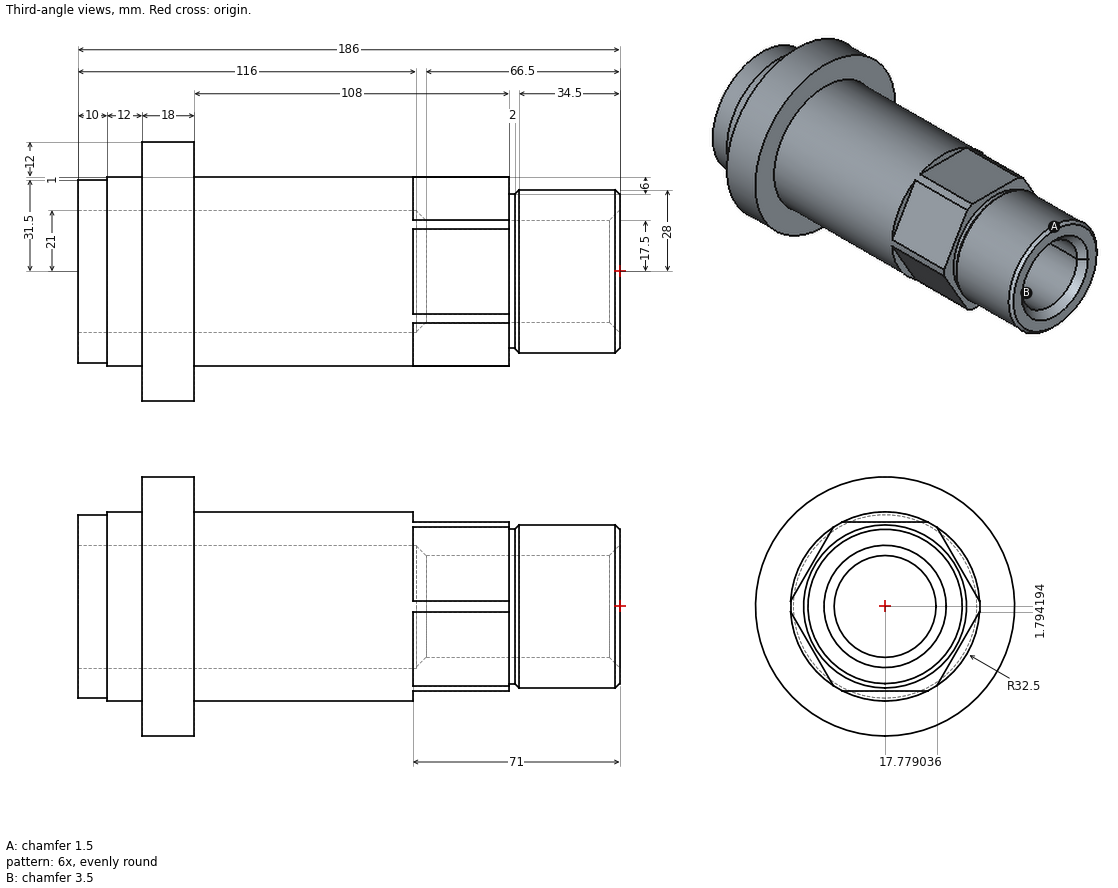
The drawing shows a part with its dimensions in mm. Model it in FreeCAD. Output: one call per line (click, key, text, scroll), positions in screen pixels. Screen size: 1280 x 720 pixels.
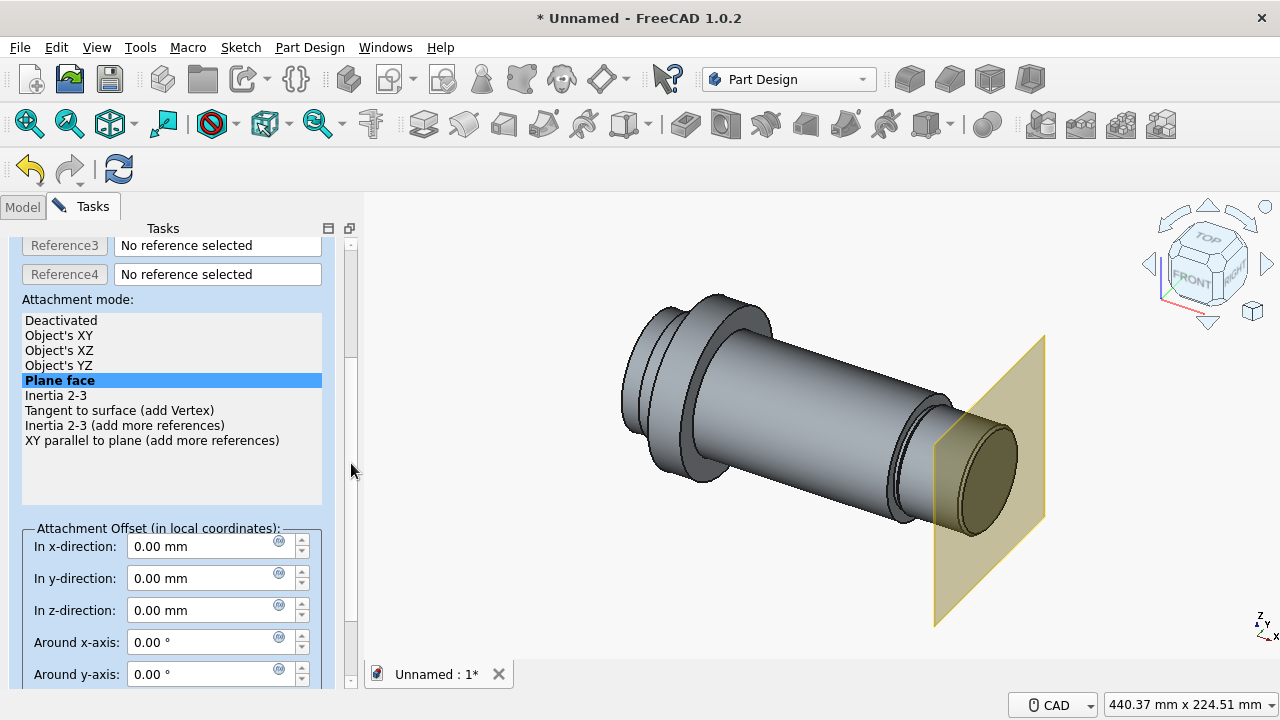
triple_click(210, 610)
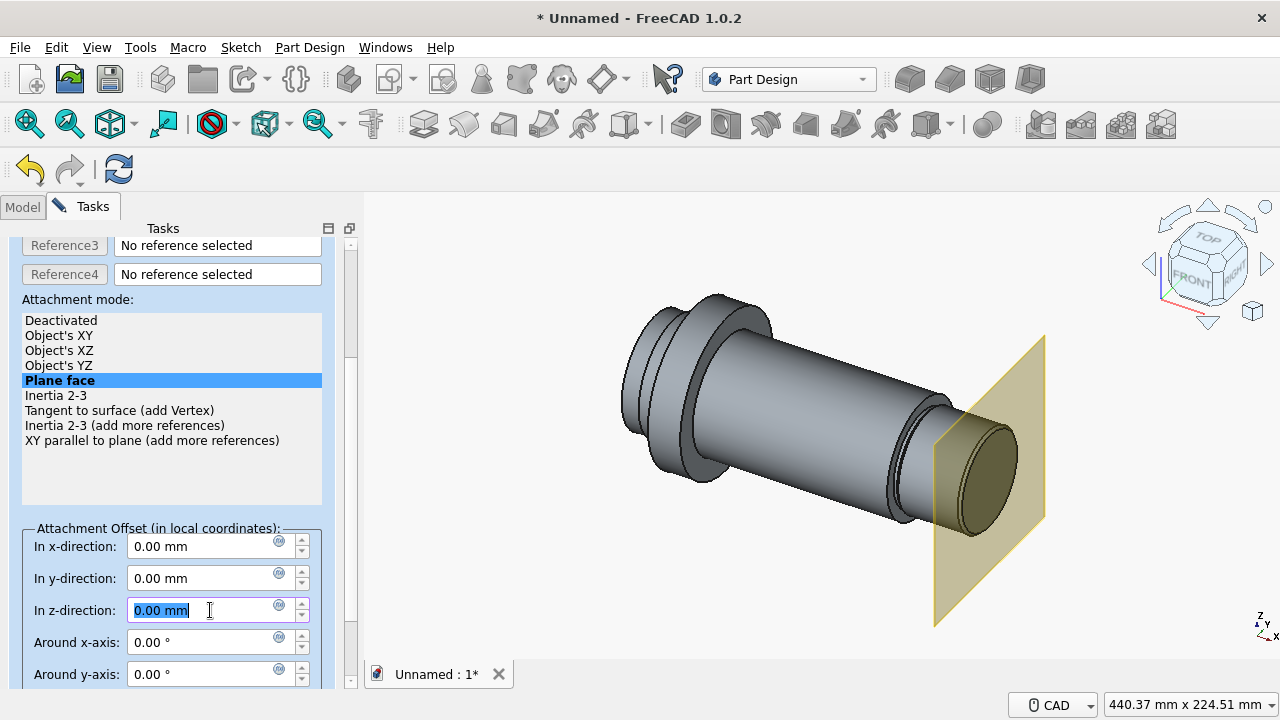
text(-71)
key(Tab)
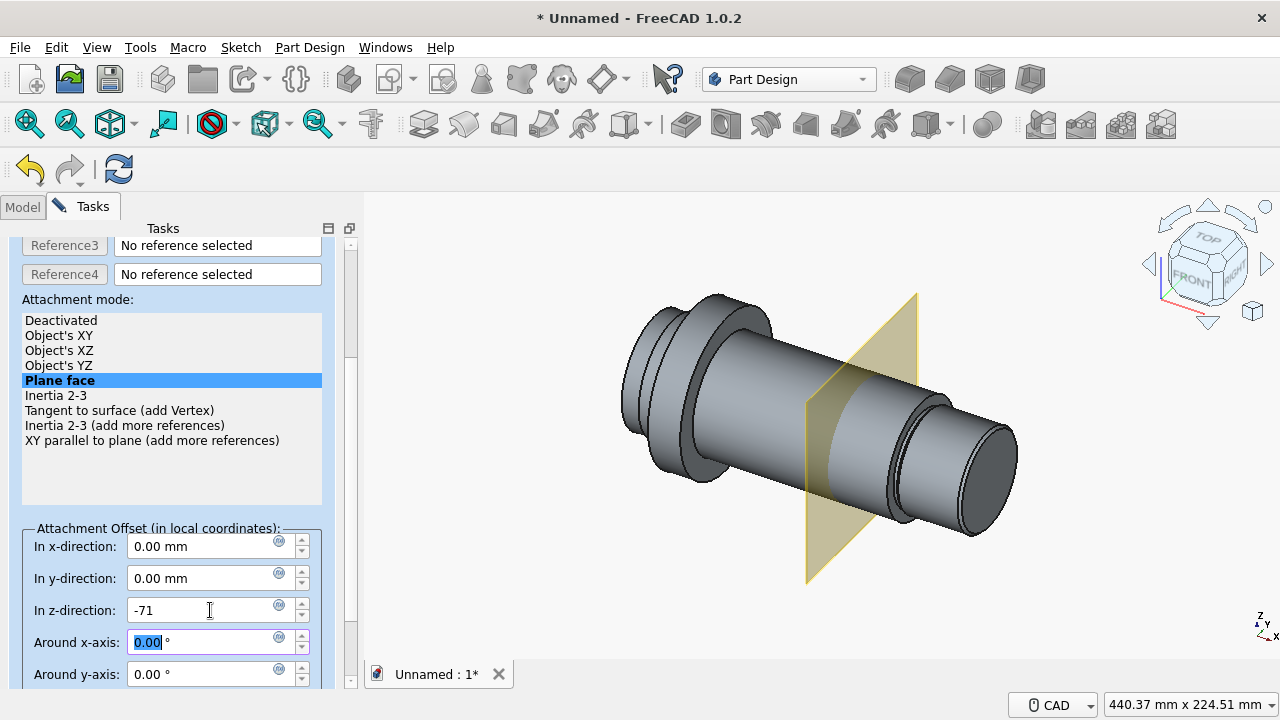
scroll(351, 463, up, 4)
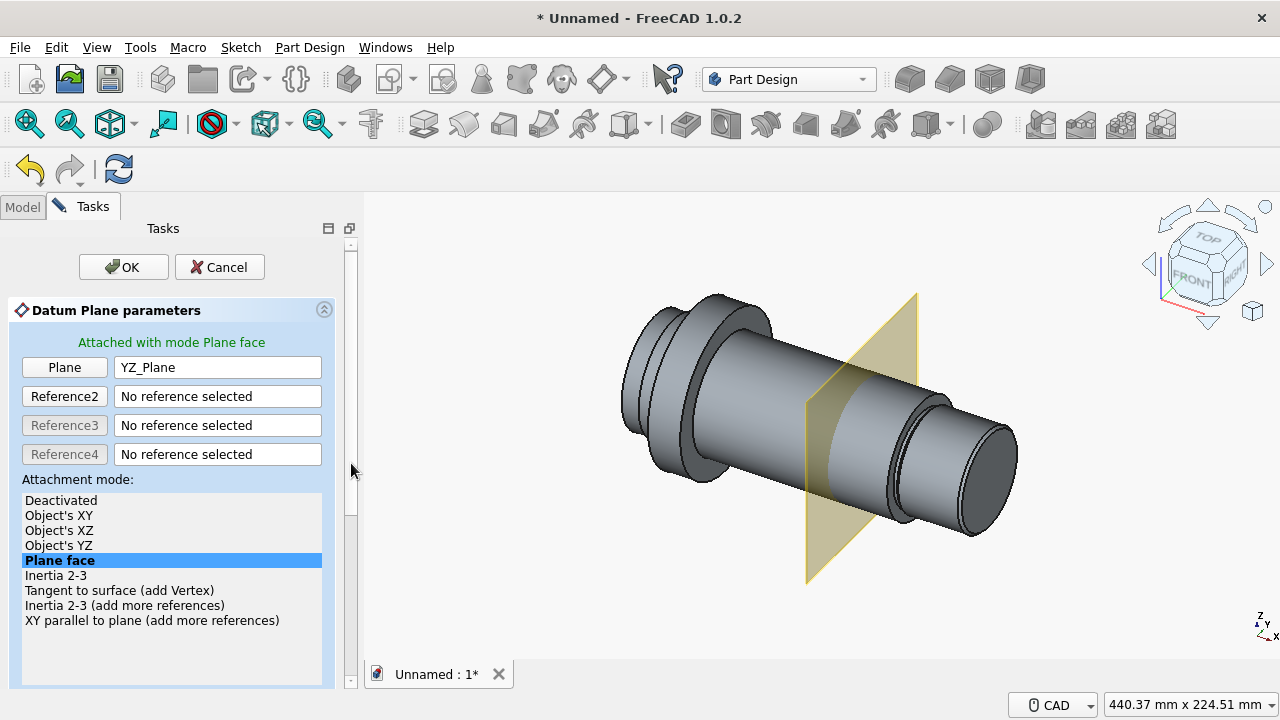
click(124, 267)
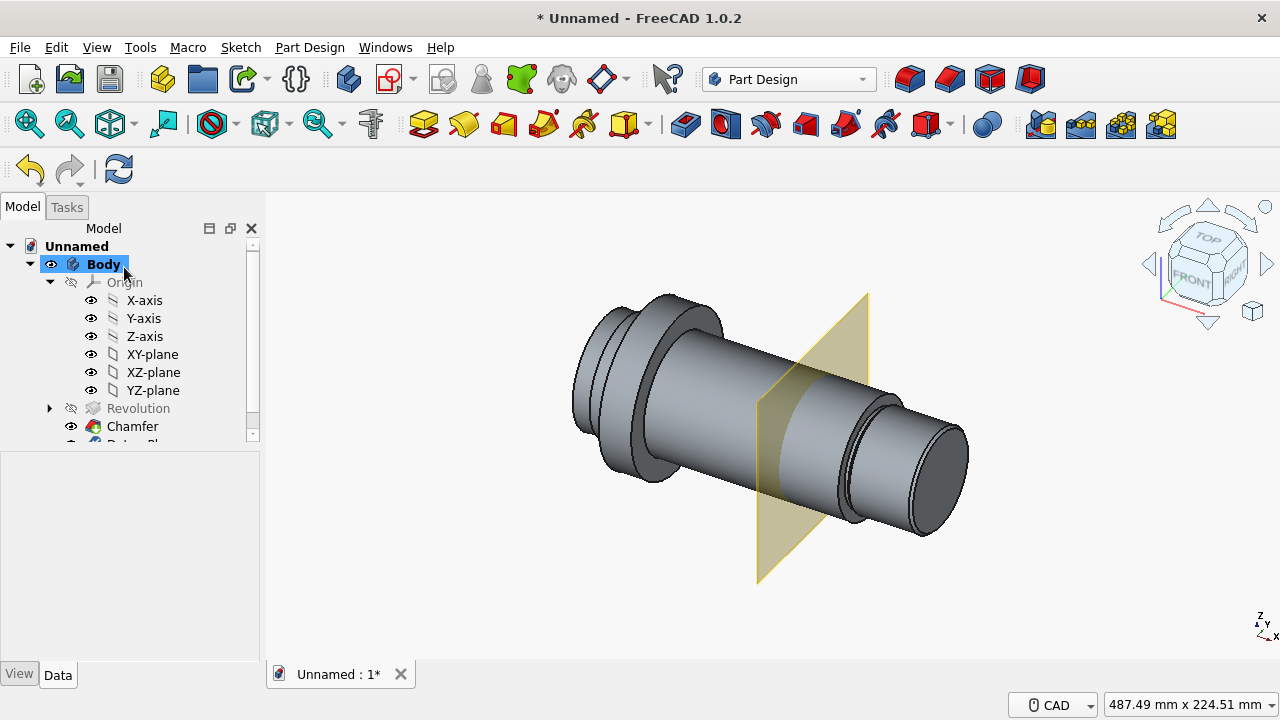
scroll(100, 332, down, 3)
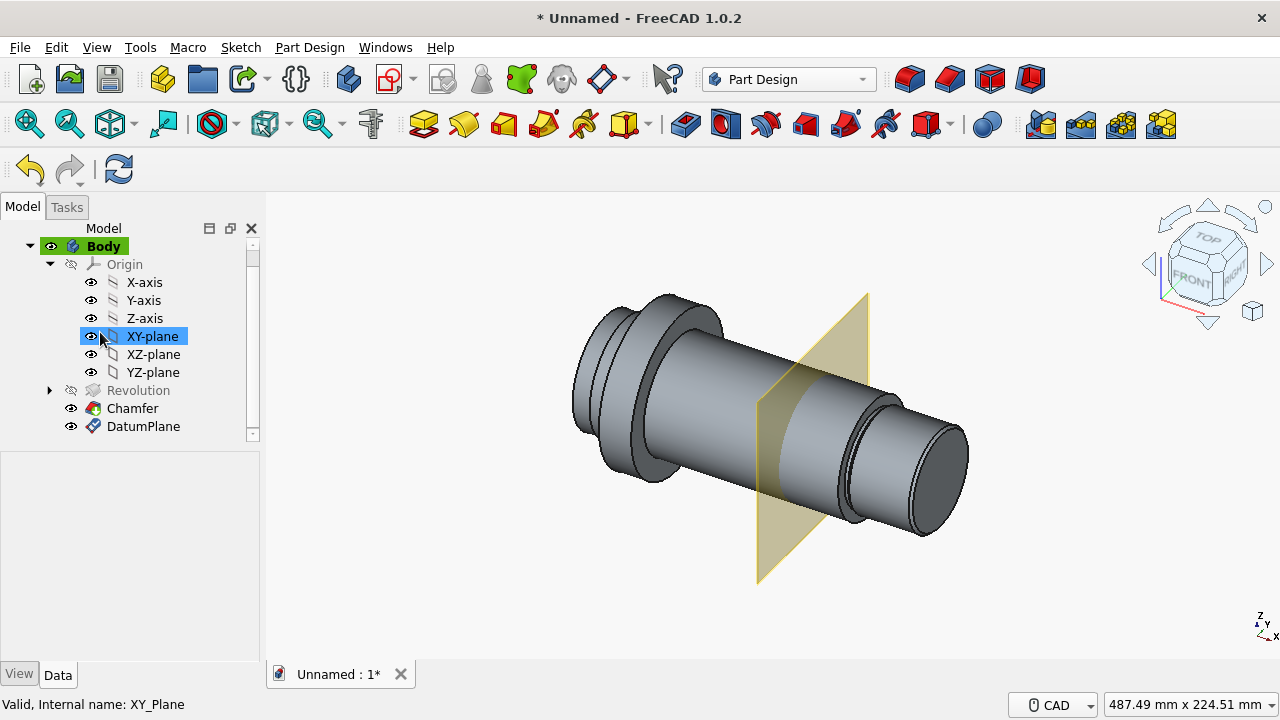
click(116, 426)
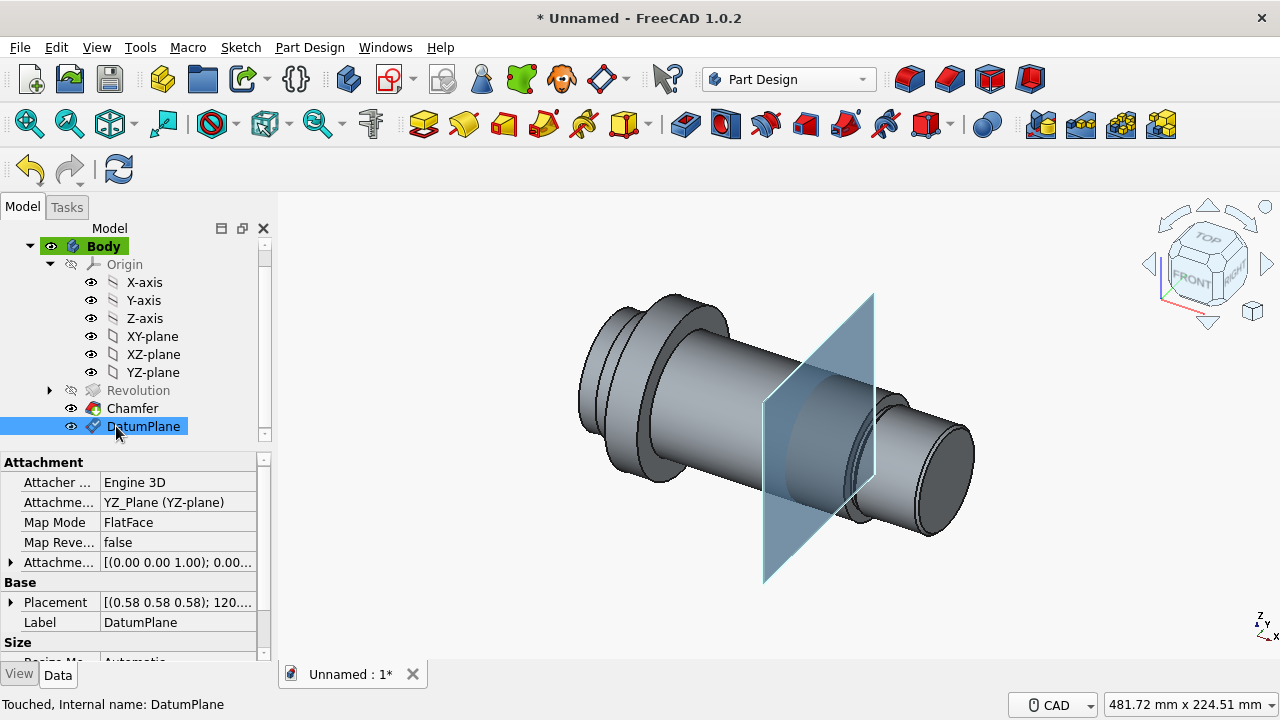
click(390, 80)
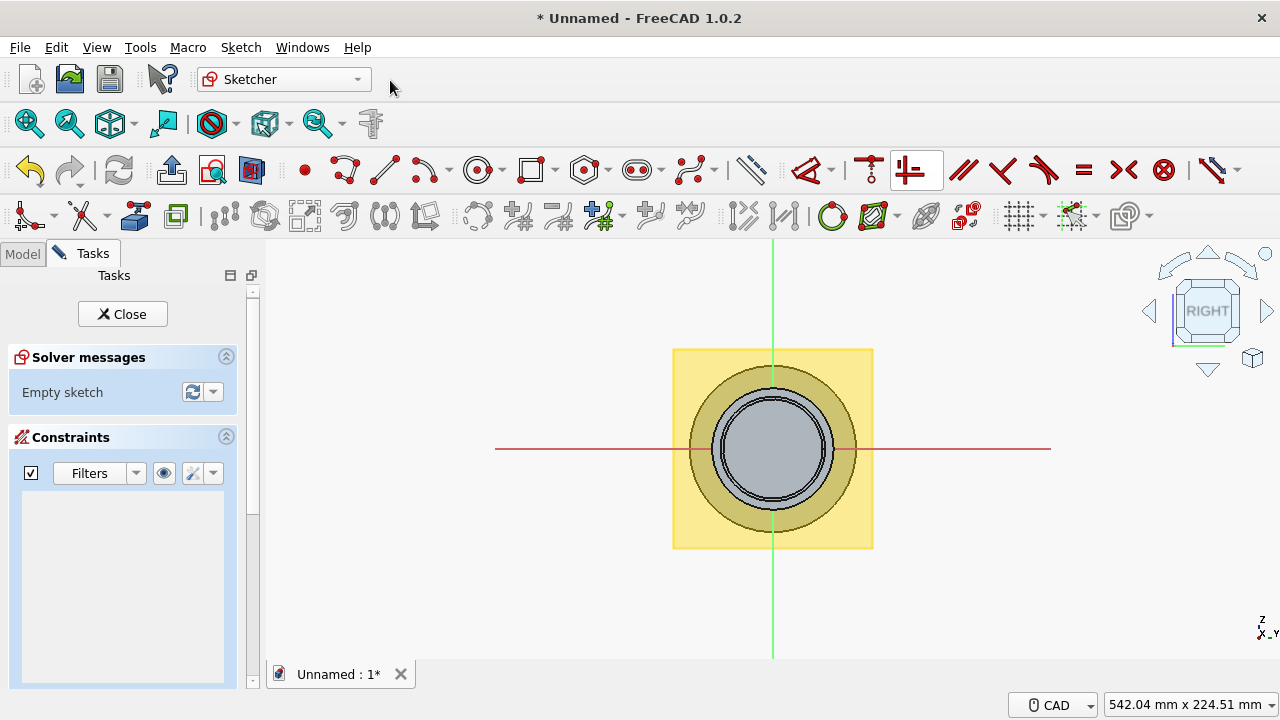
click(252, 170)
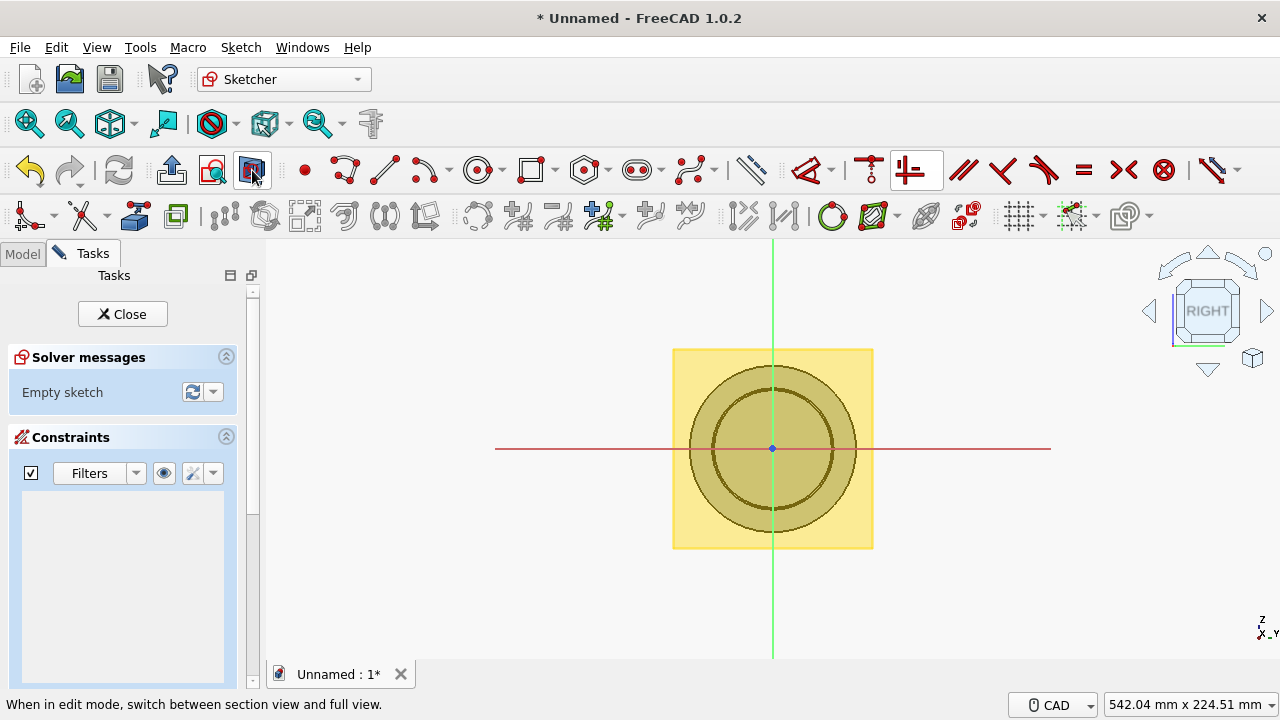
scroll(828, 481, up, 8)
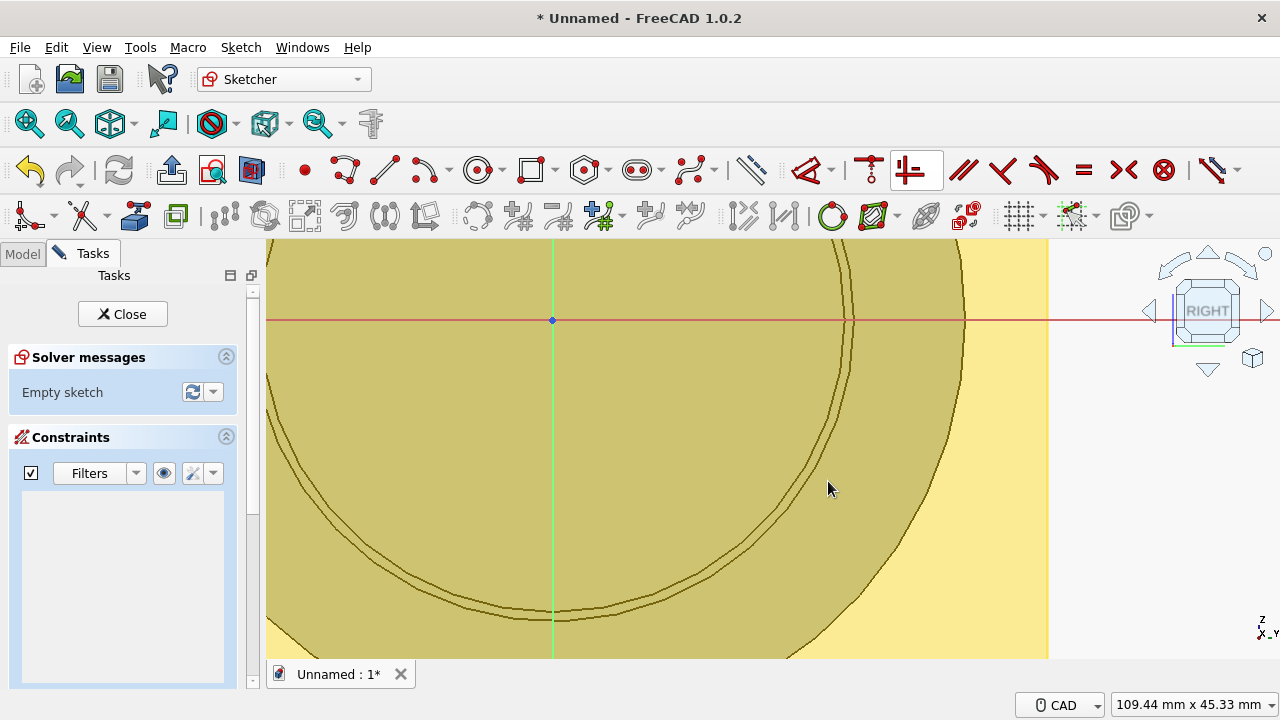
click(386, 170)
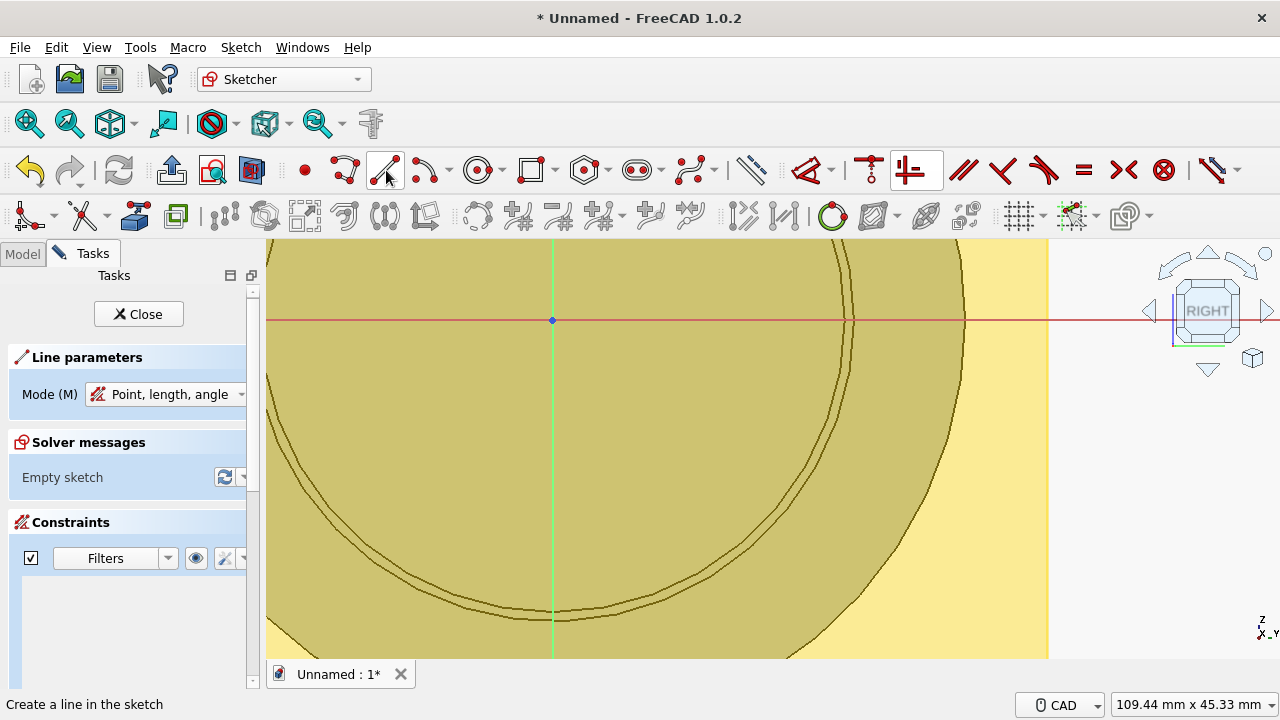
click(854, 337)
click(718, 572)